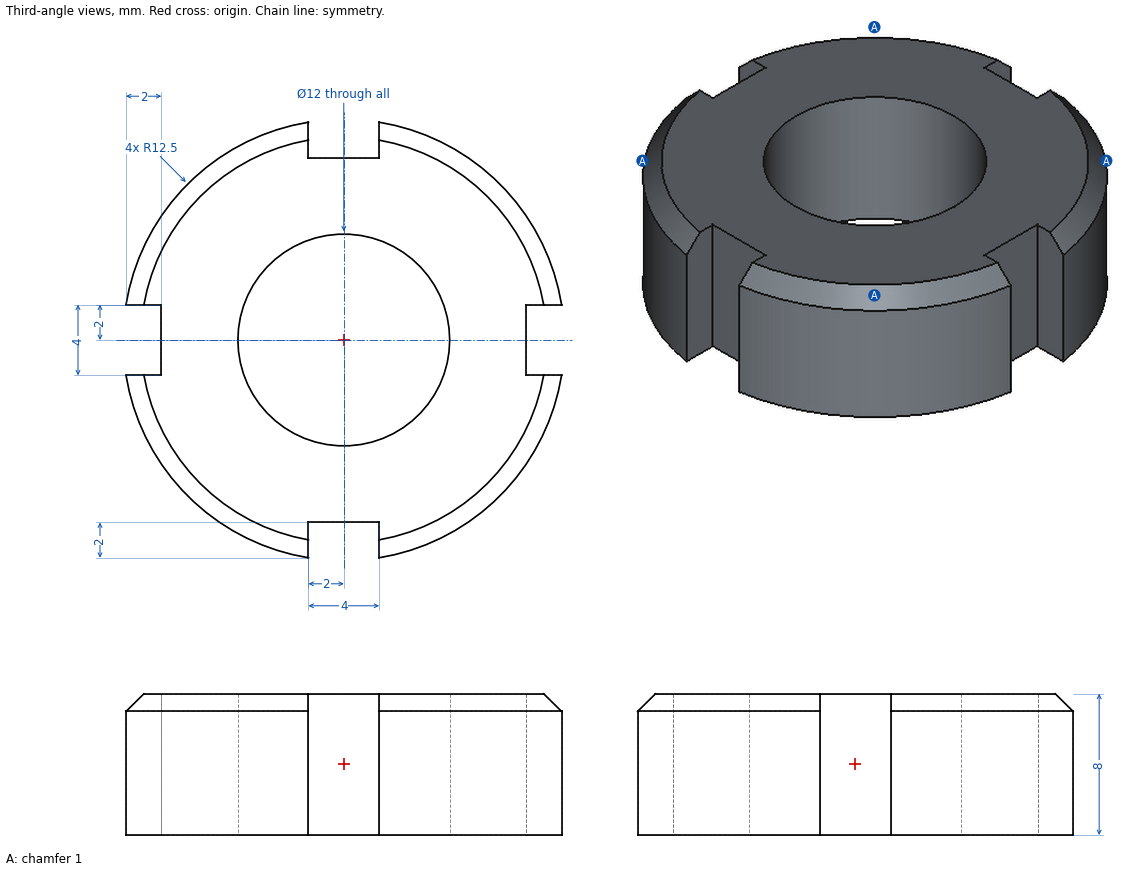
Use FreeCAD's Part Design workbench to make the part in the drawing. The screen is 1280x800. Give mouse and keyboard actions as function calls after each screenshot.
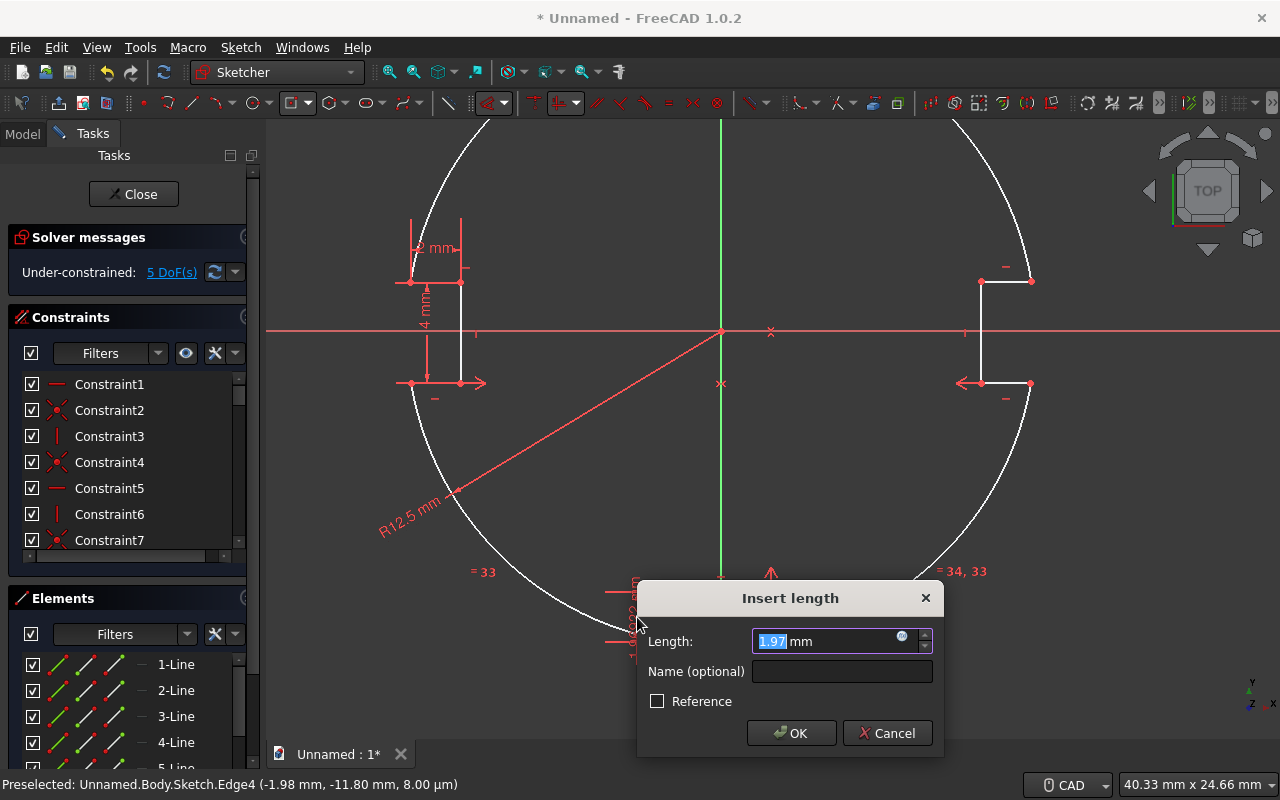
text(2)
key(Return)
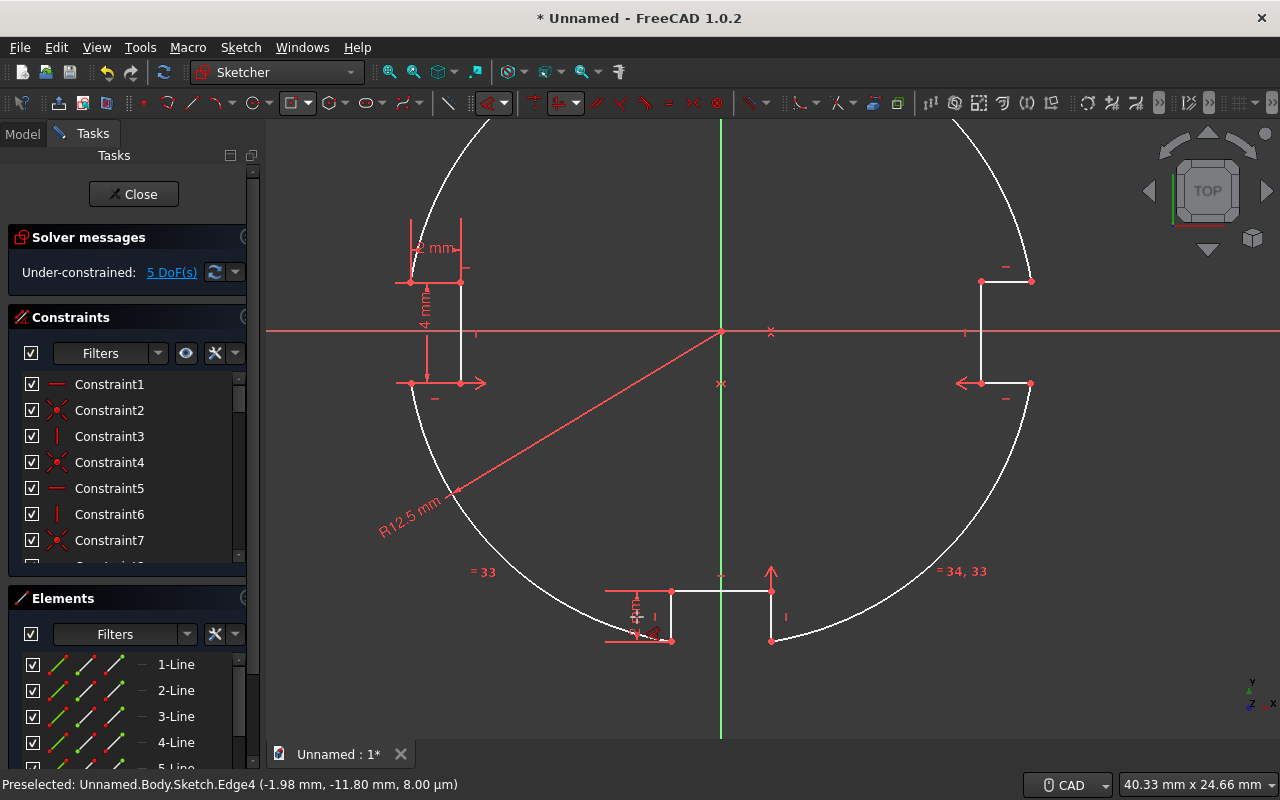
click(701, 591)
click(744, 625)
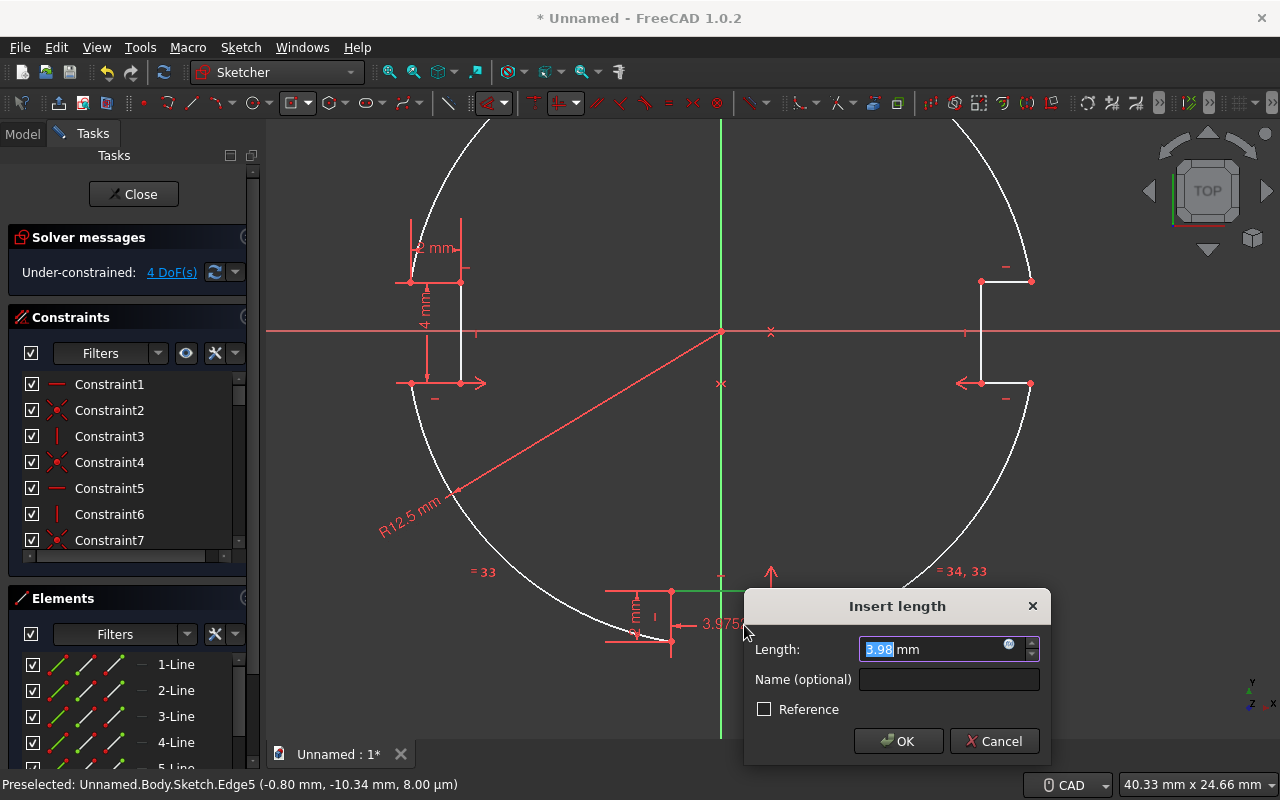
text(4)
key(Return)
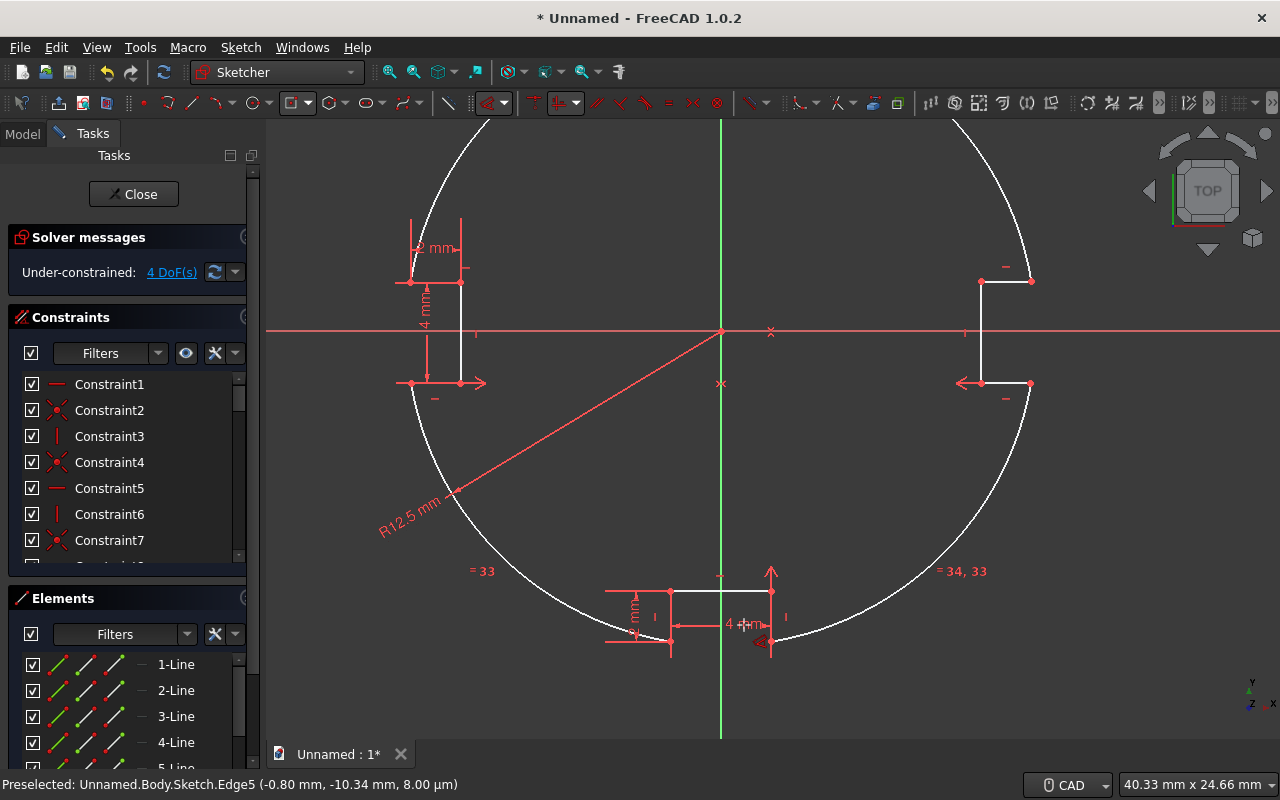
click(981, 353)
click(1015, 309)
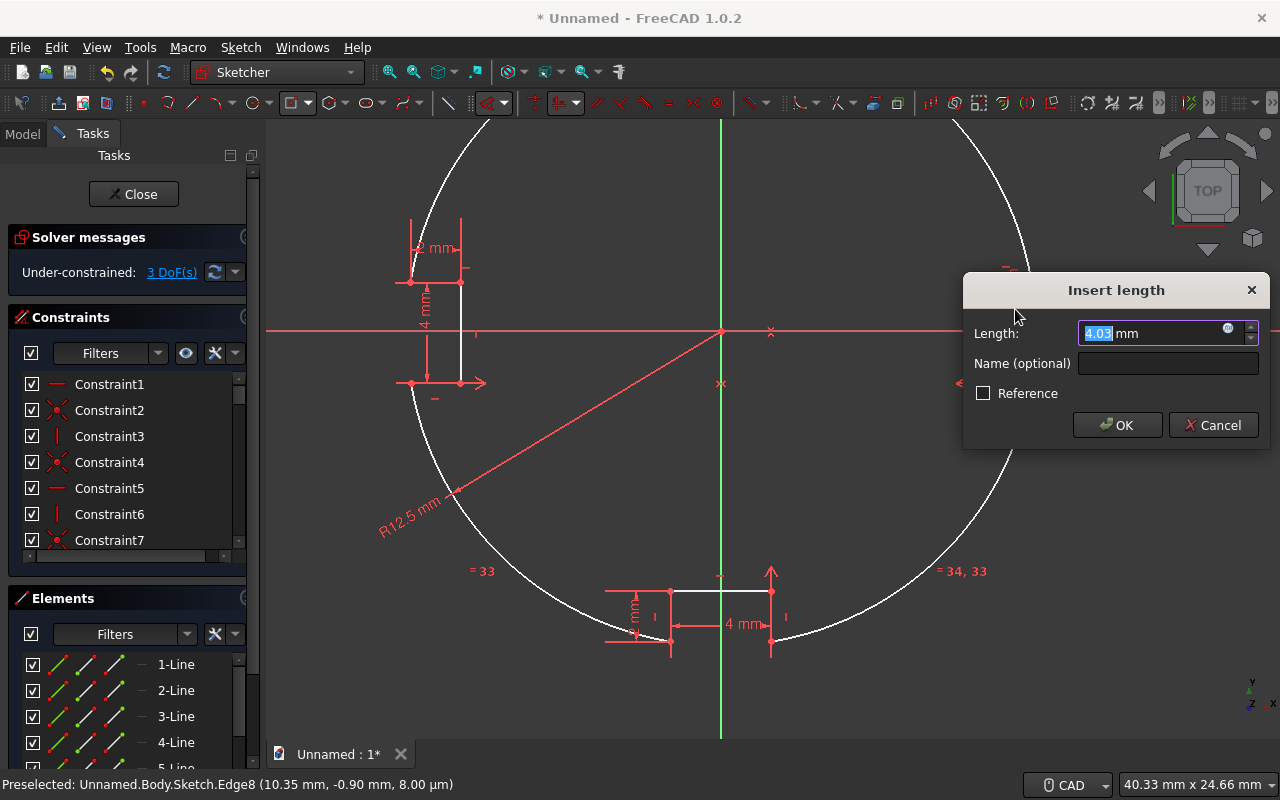
text(4)
key(Return)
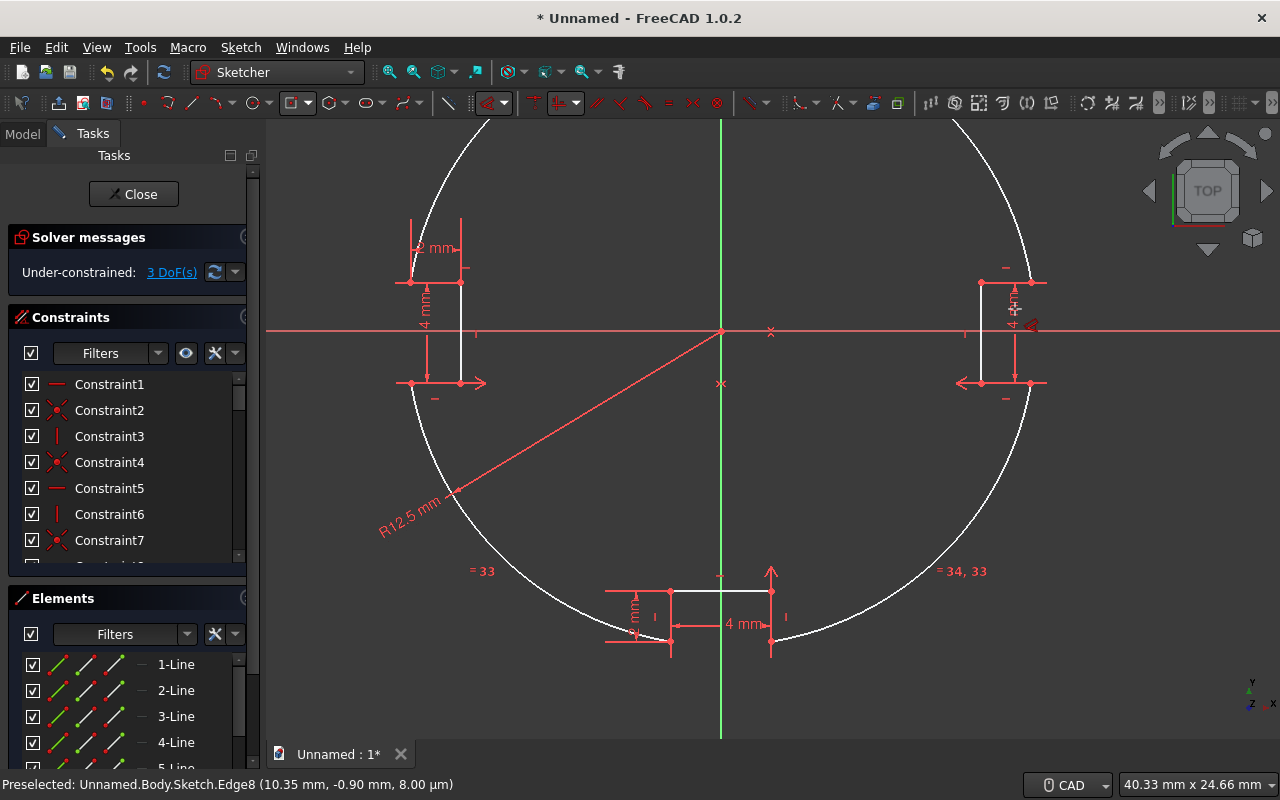
scroll(671, 627, down, 2)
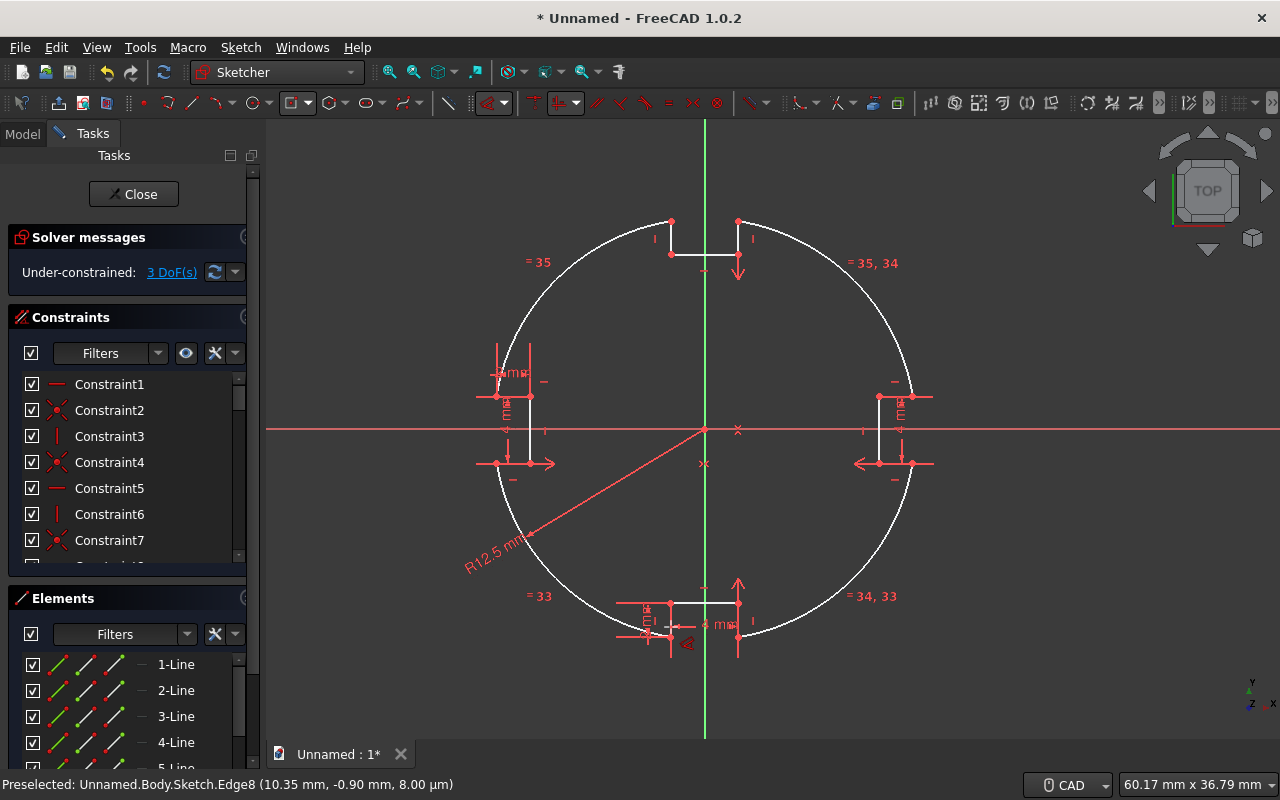
click(718, 255)
click(689, 221)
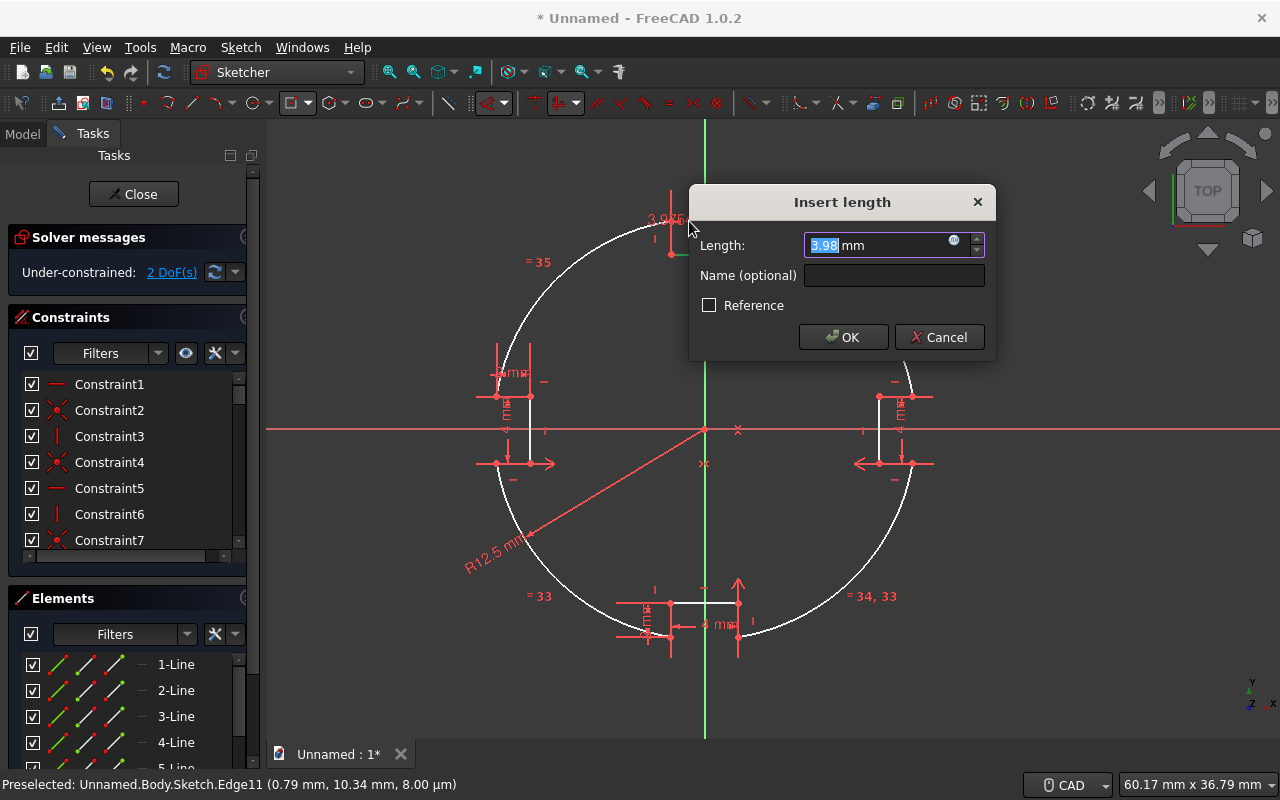
text(4)
key(Return)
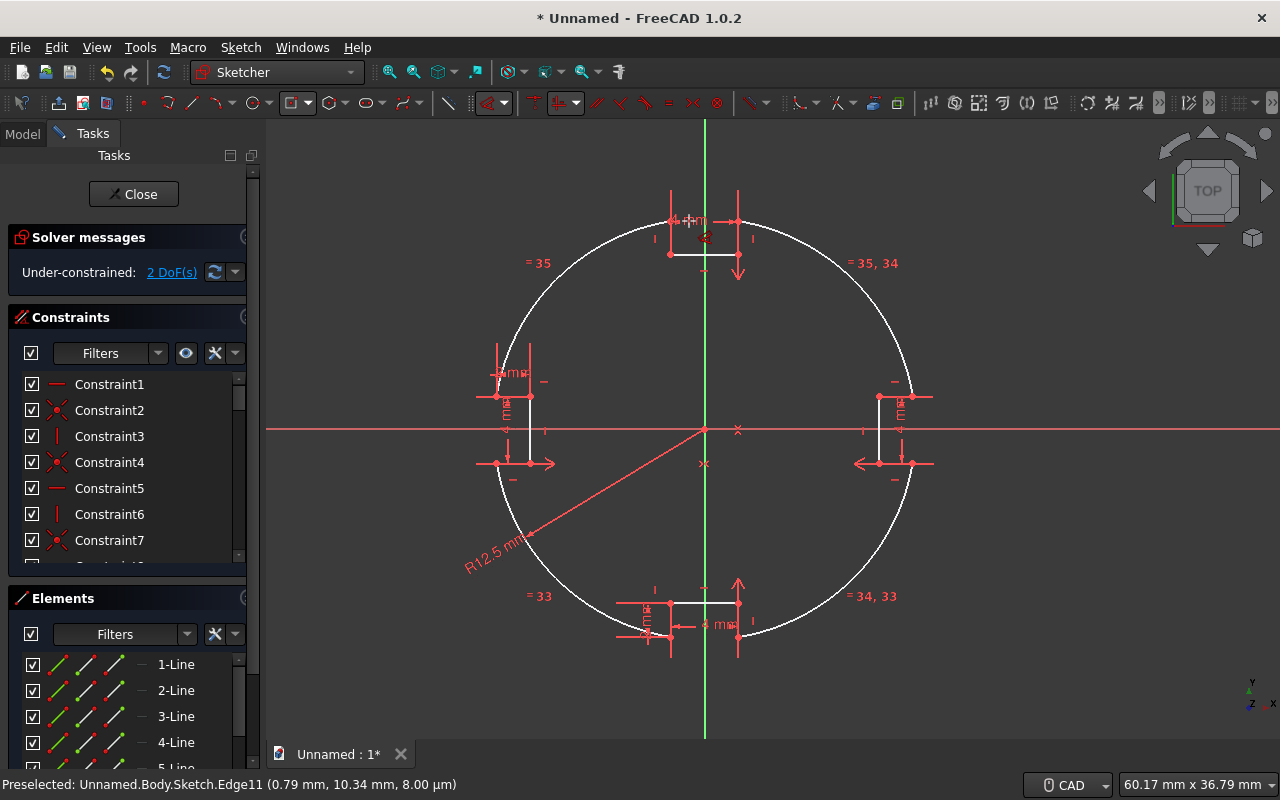
click(497, 397)
click(739, 413)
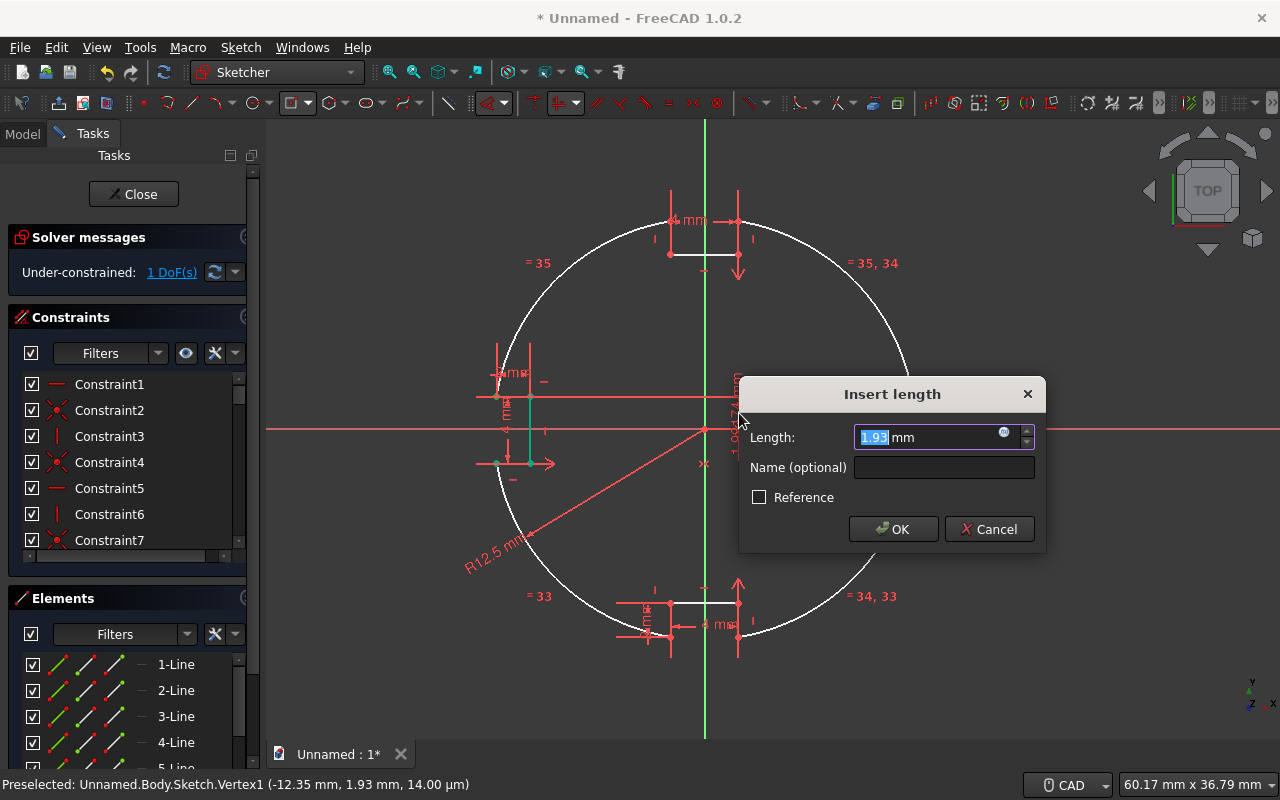
text(2)
key(Return)